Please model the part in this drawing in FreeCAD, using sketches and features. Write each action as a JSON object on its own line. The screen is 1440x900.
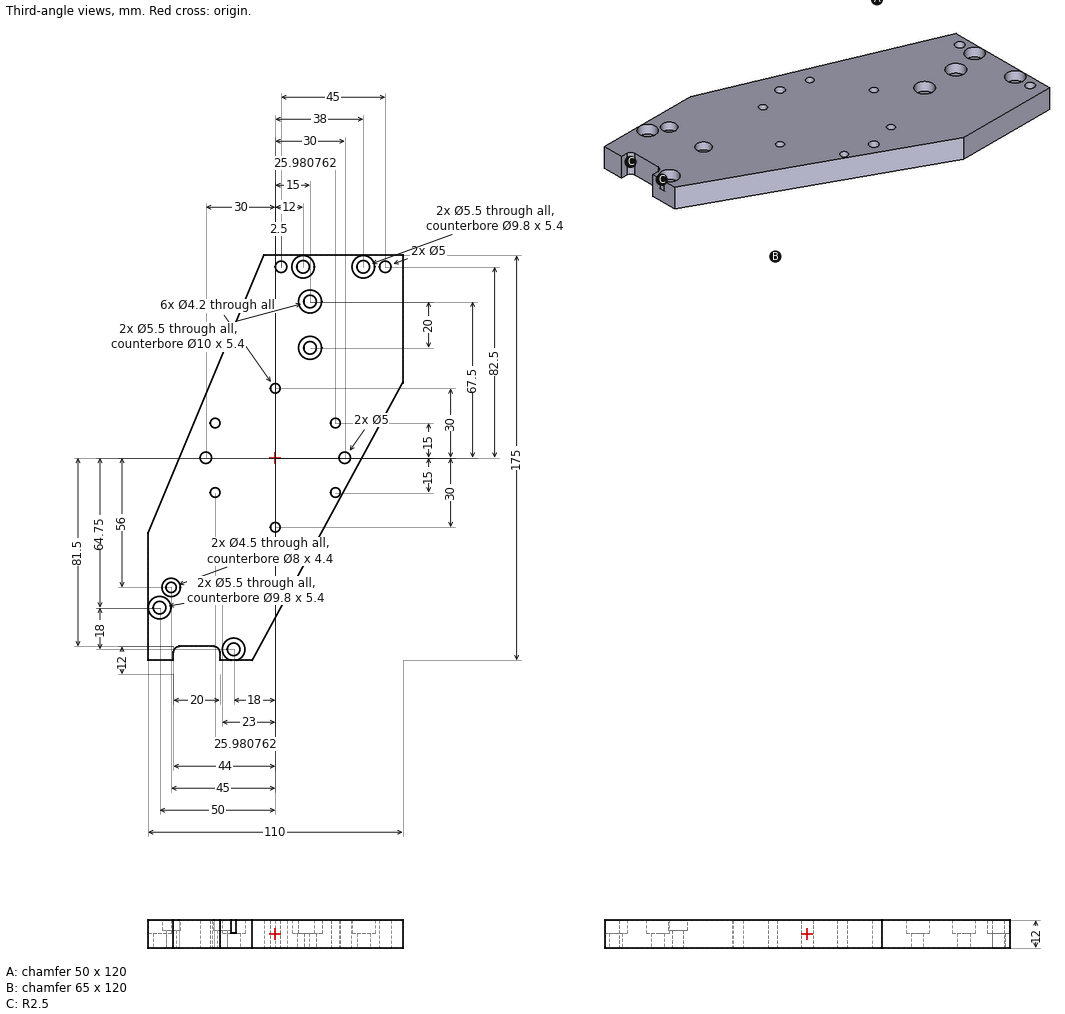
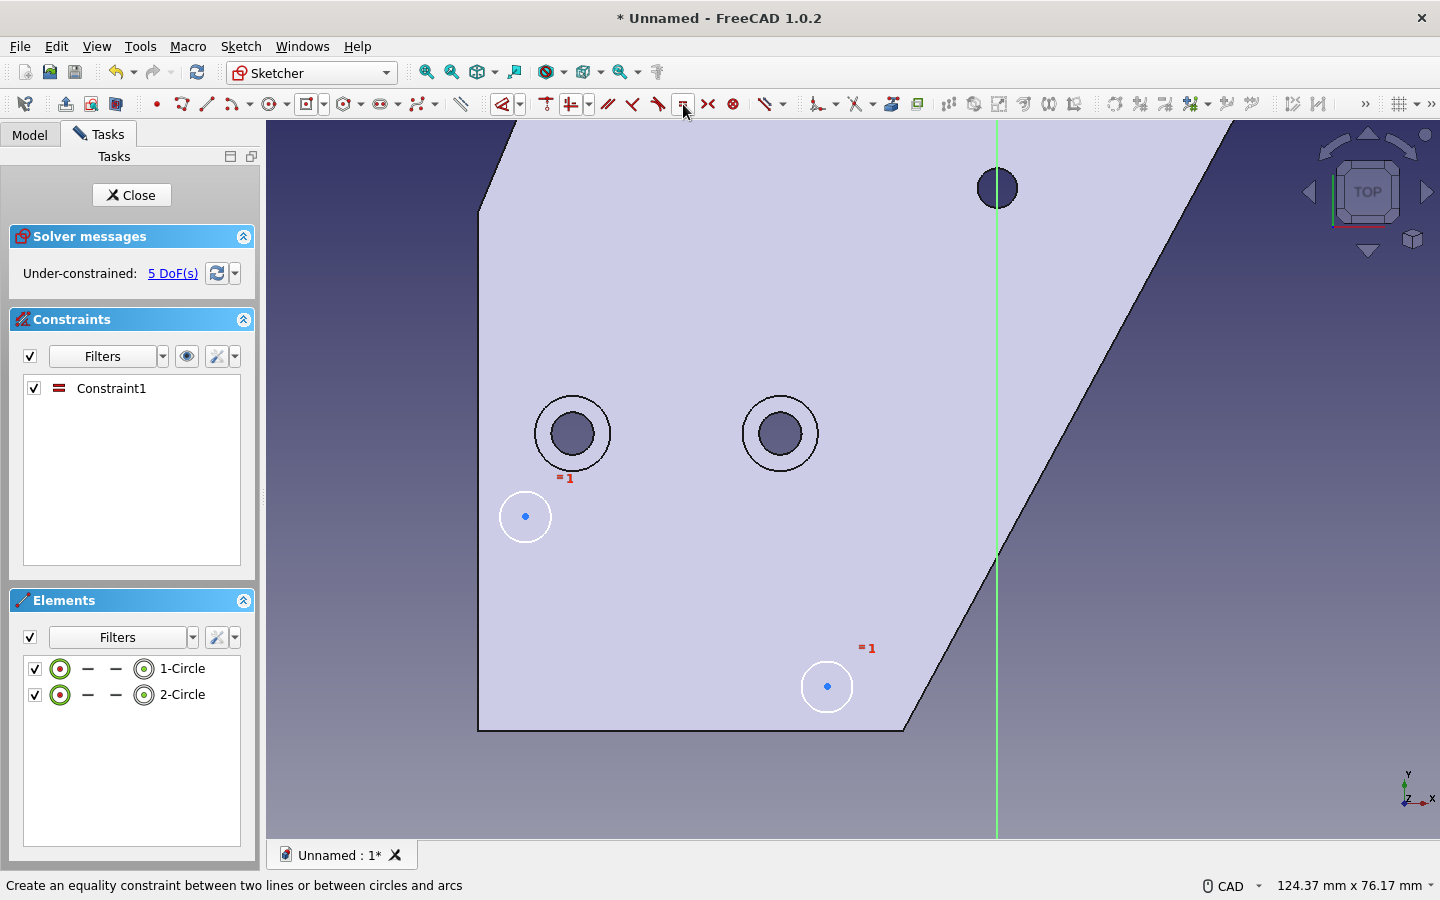
{"action": "left_click", "coordinate": [543, 499]}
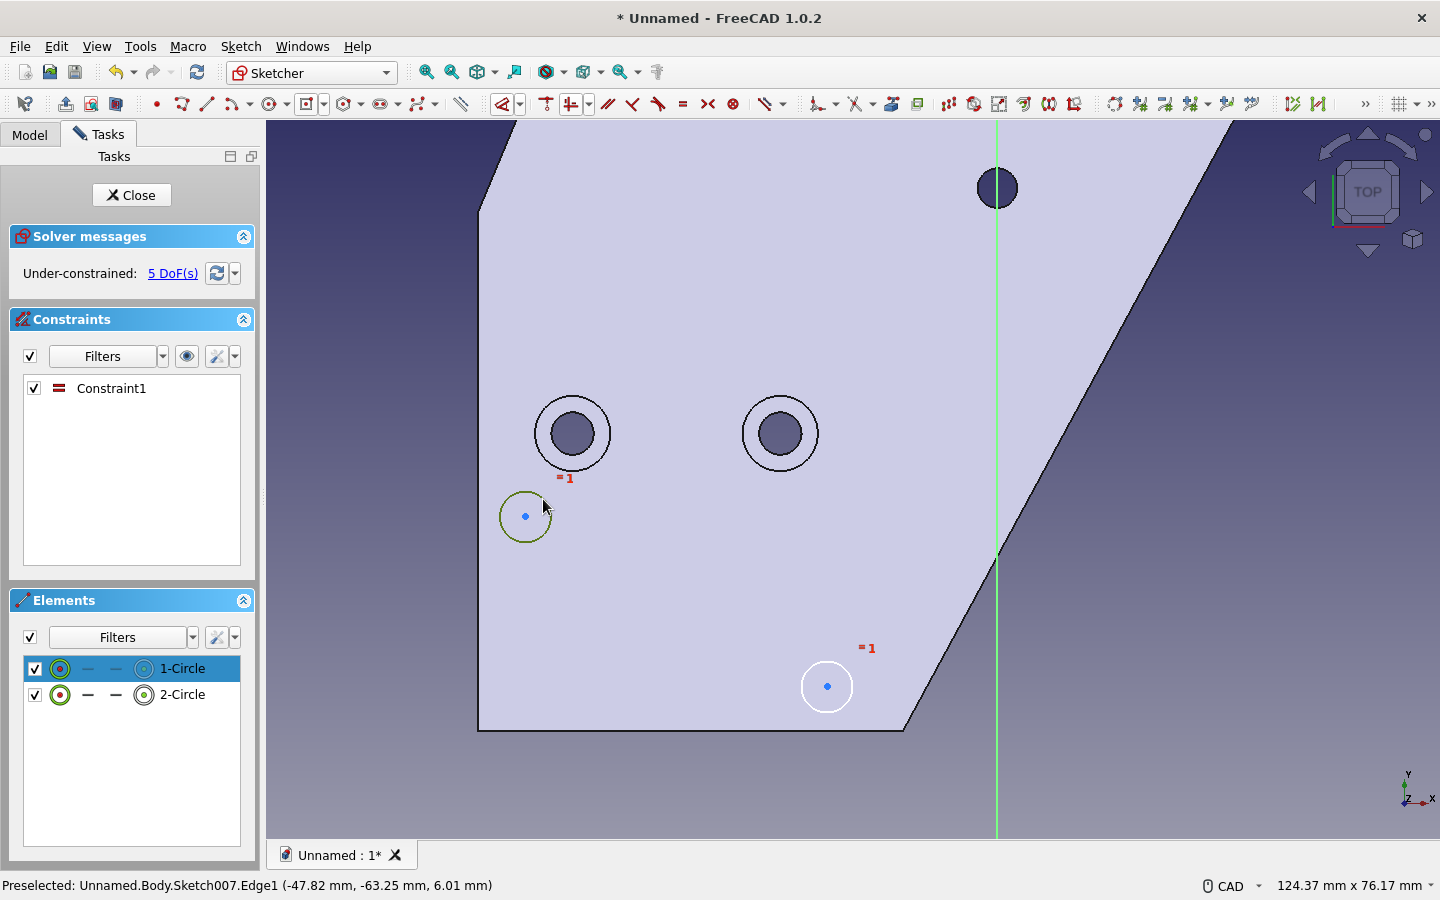
{"action": "key", "text": "k o"}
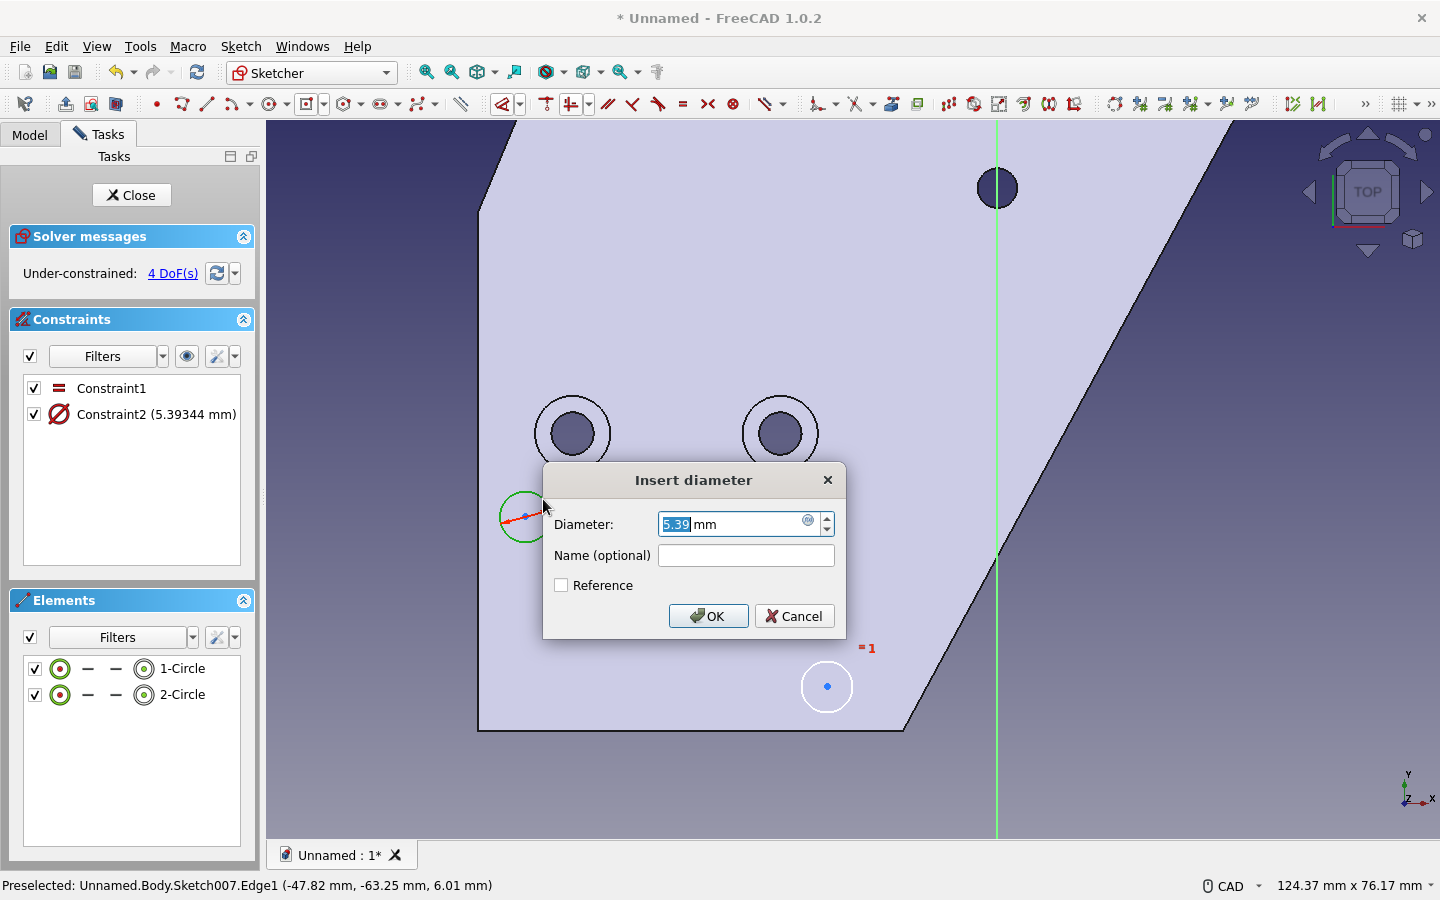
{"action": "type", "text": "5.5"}
{"action": "key", "text": "Return"}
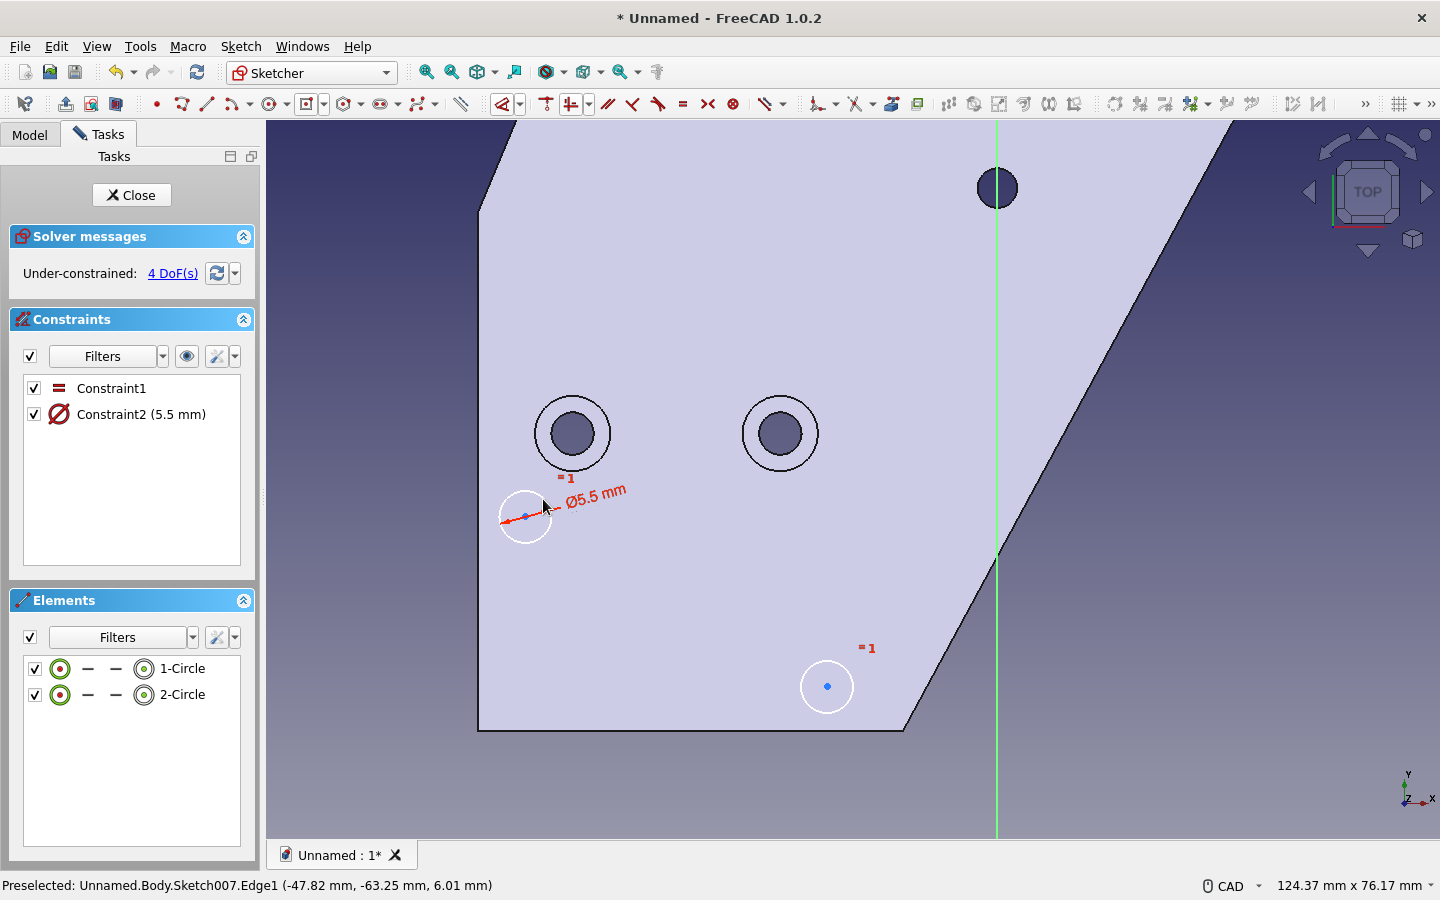
{"action": "left_click", "coordinate": [525, 517]}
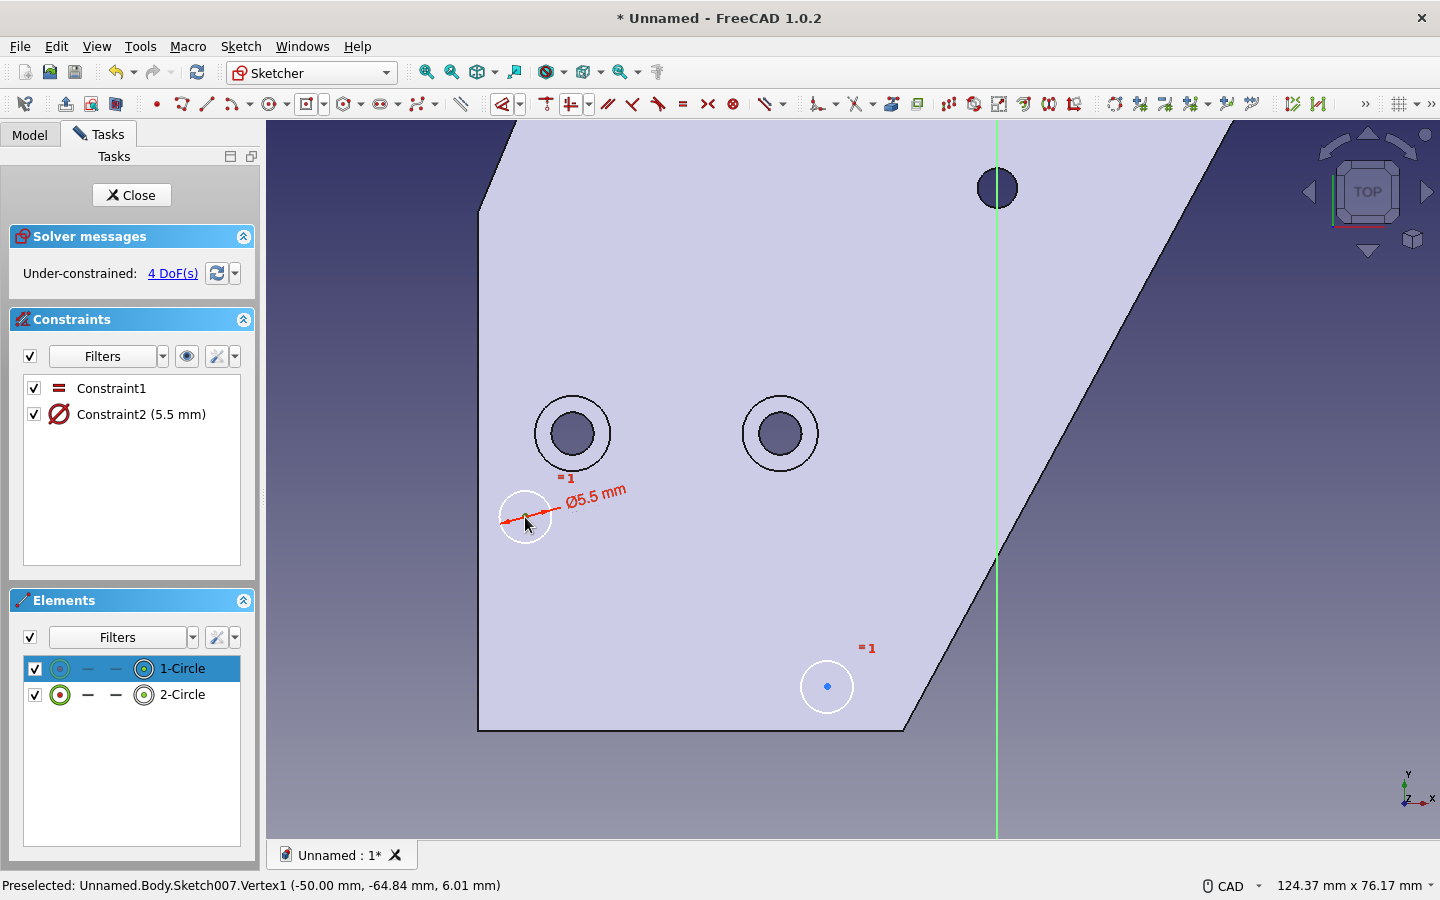
{"action": "key", "text": "l"}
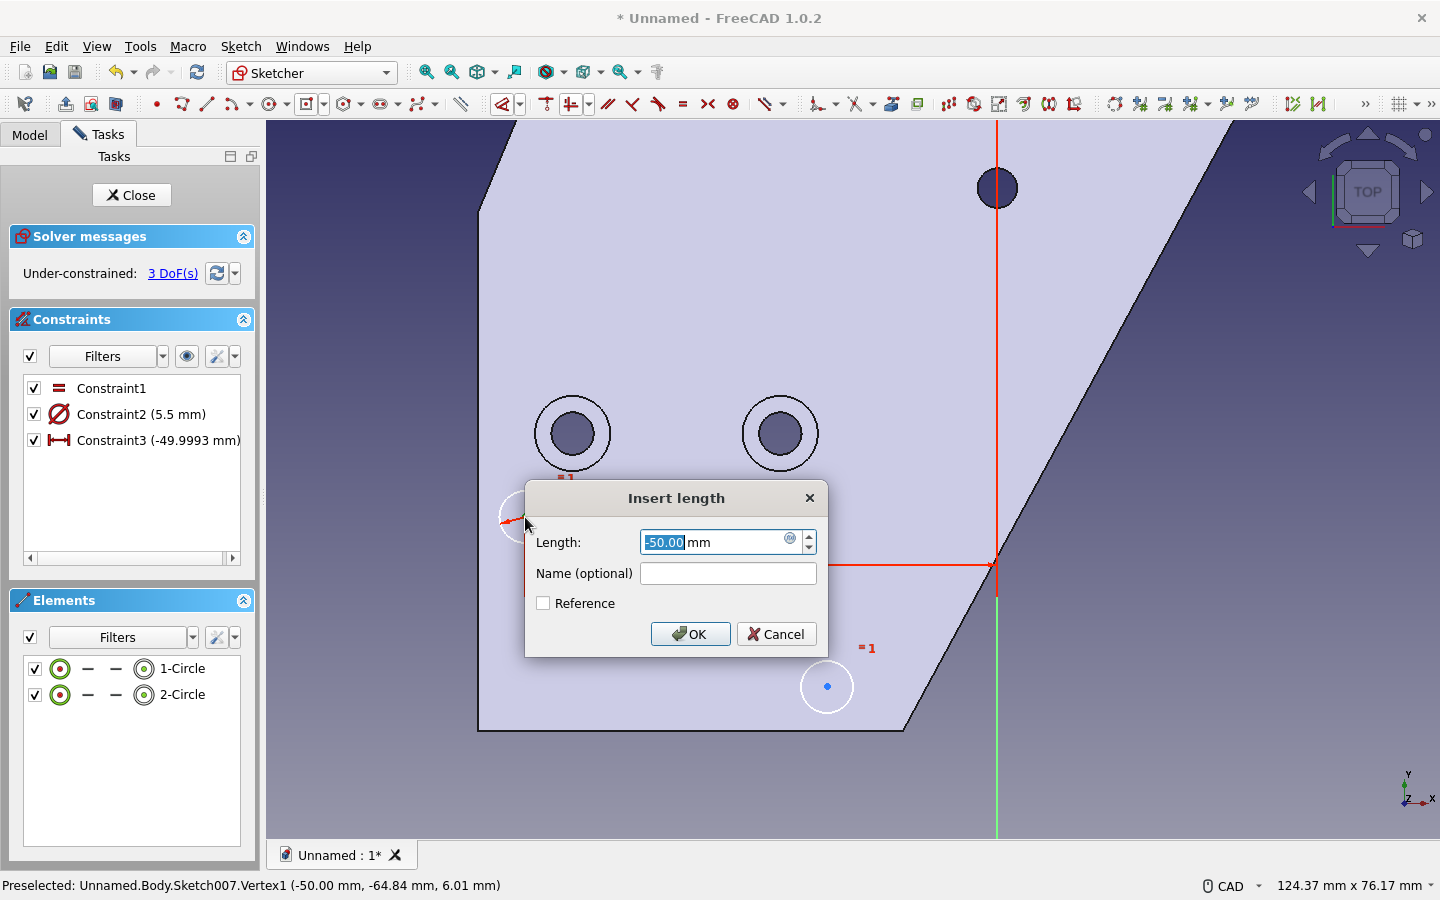
{"action": "type", "text": "-50"}
{"action": "key", "text": "Return"}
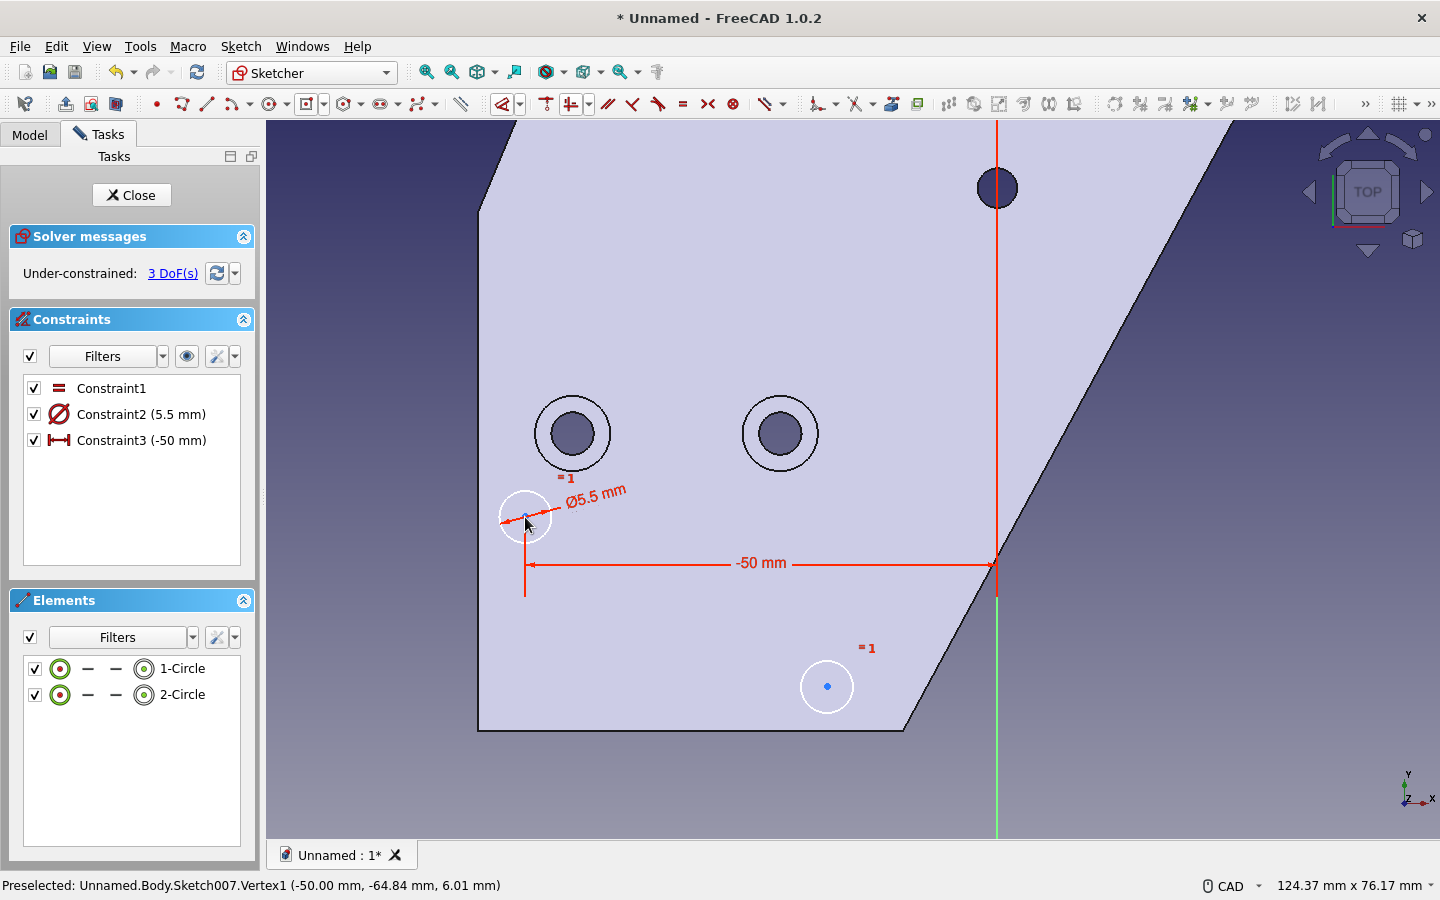
{"action": "left_click", "coordinate": [827, 687]}